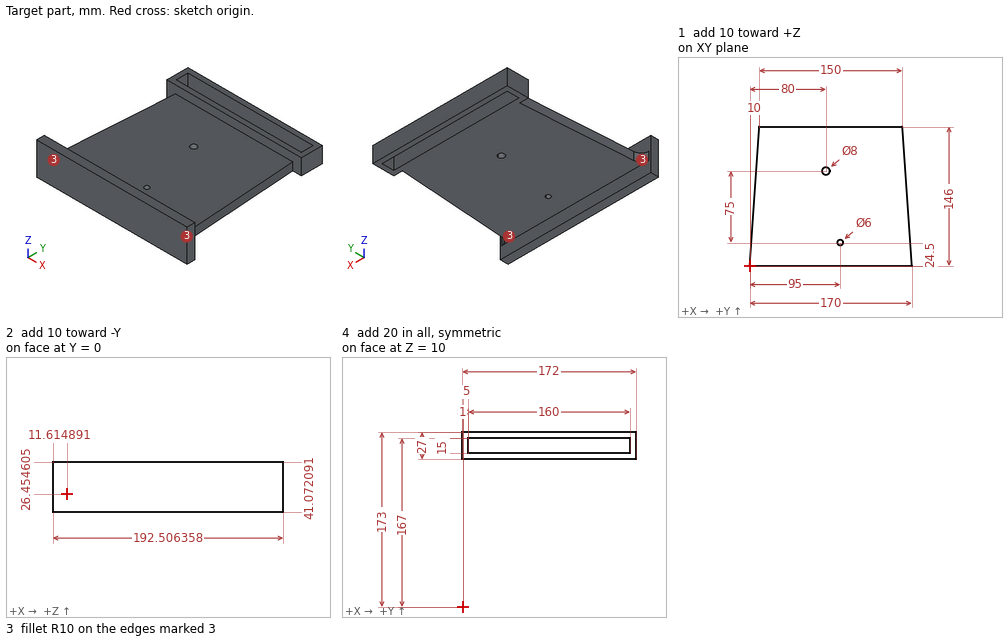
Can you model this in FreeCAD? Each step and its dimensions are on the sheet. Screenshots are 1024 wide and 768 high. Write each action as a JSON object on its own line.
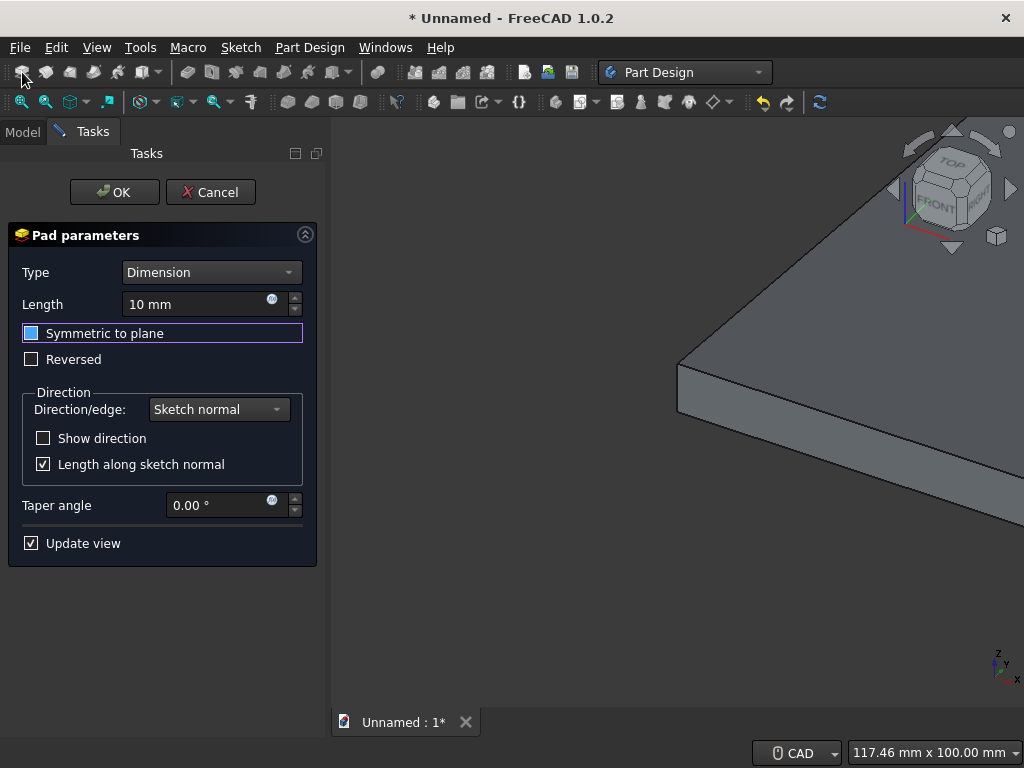
{"action": "left_click", "coordinate": [115, 192]}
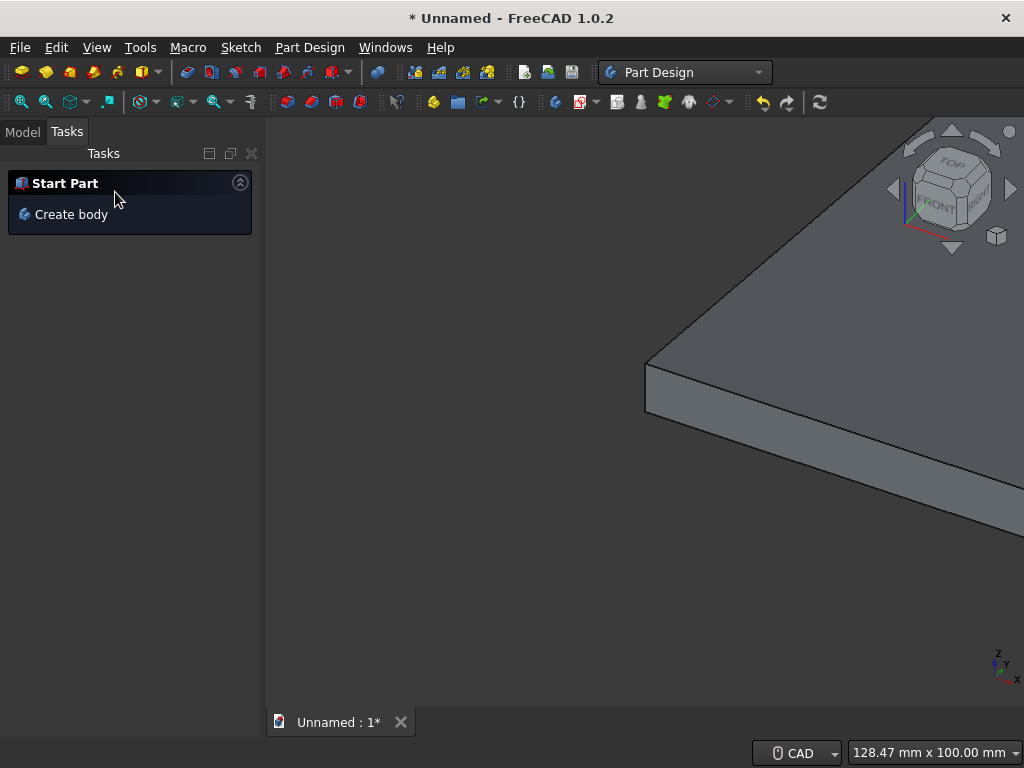
{"action": "key", "text": "v f"}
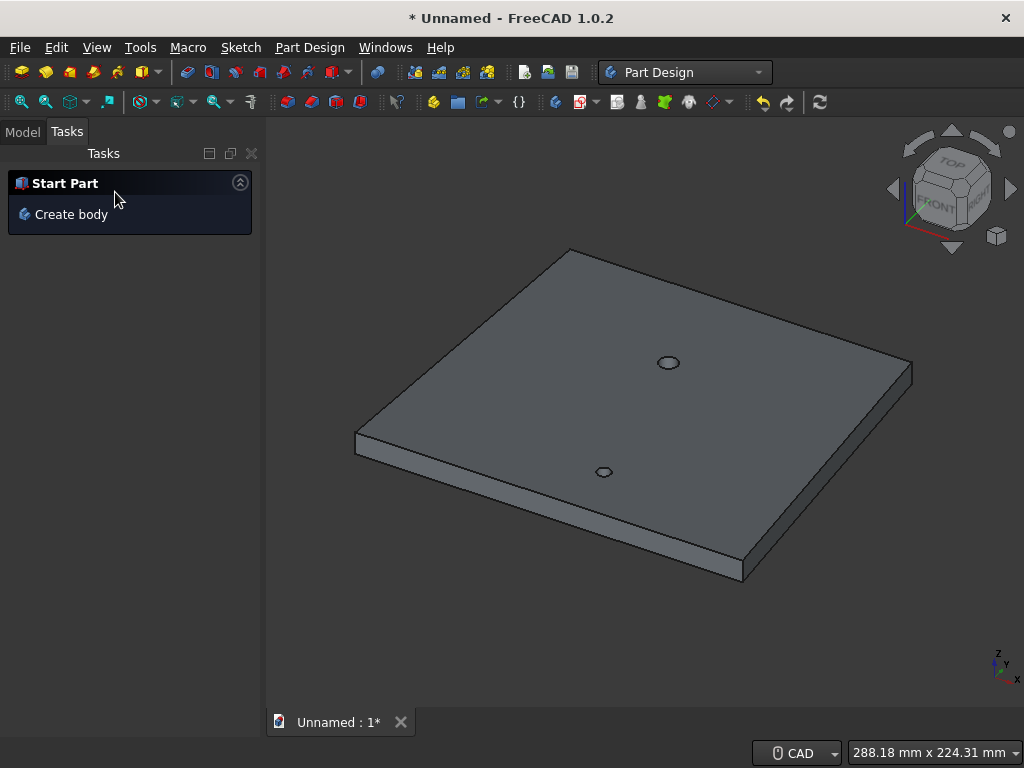
{"action": "left_click", "coordinate": [715, 561]}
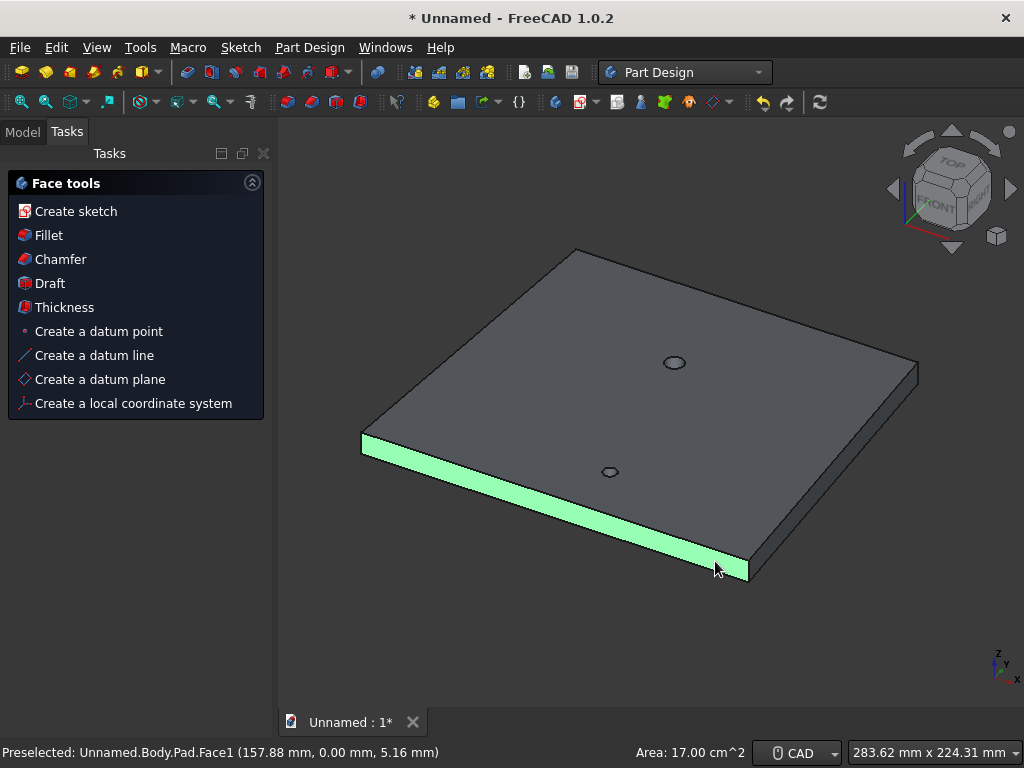
{"action": "left_click", "coordinate": [580, 102]}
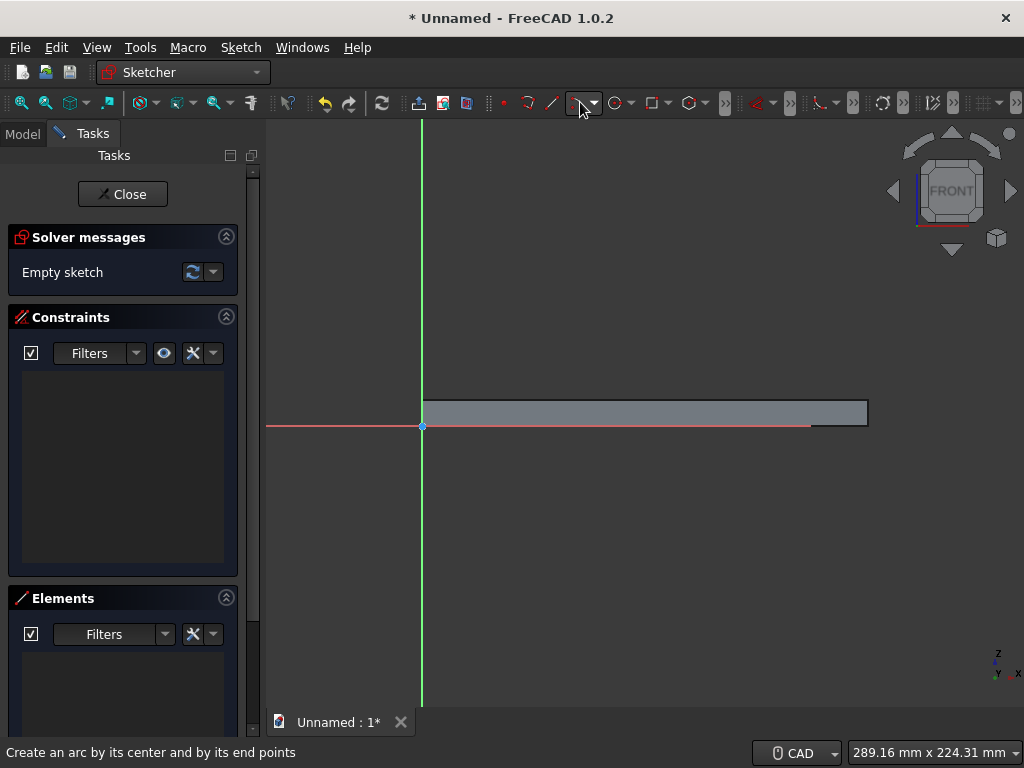
{"action": "scroll", "coordinate": [294, 424], "scroll_direction": "down", "scroll_amount": 1}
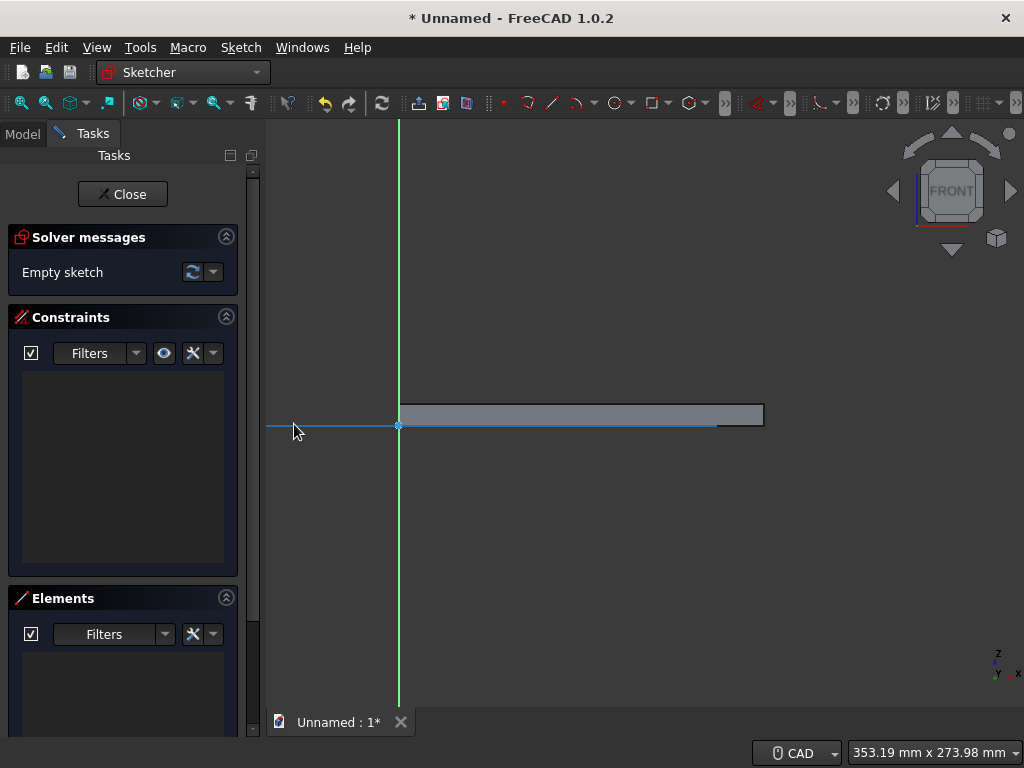
{"action": "key", "text": "g r"}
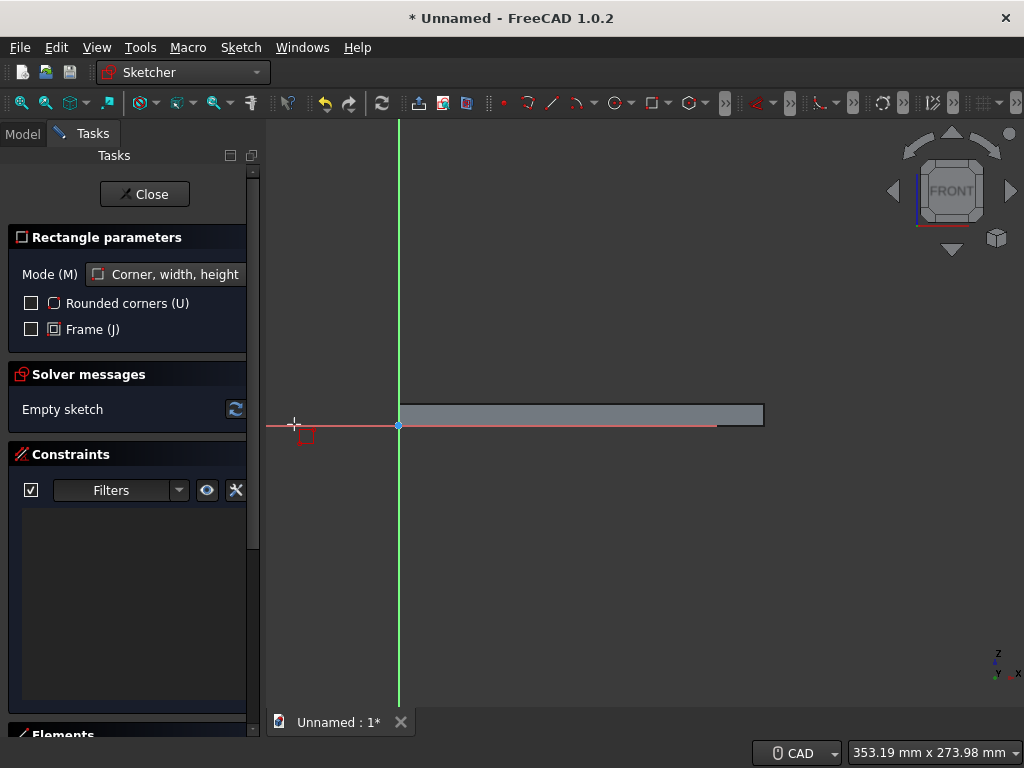
{"action": "left_click", "coordinate": [374, 369]}
{"action": "mouse_move", "coordinate": [787, 457]}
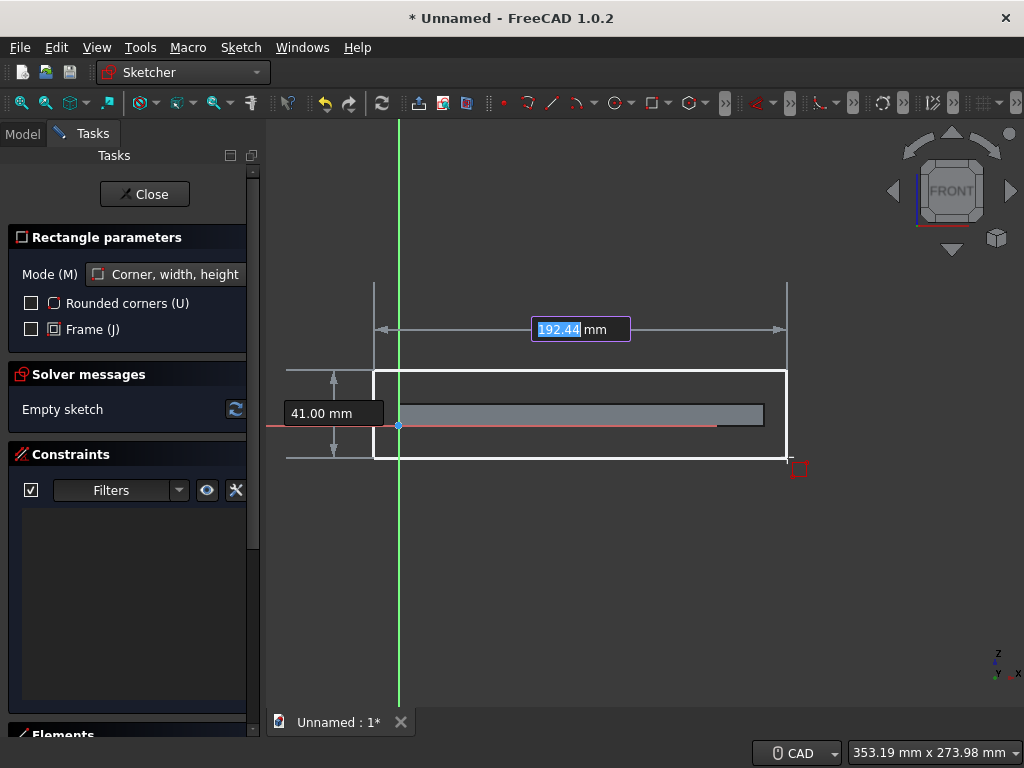
{"action": "type", "text": "192.506358"}
{"action": "key", "text": "Tab"}
{"action": "type", "text": "41.072091"}
{"action": "key", "text": "Return"}
{"action": "key", "text": "Escape"}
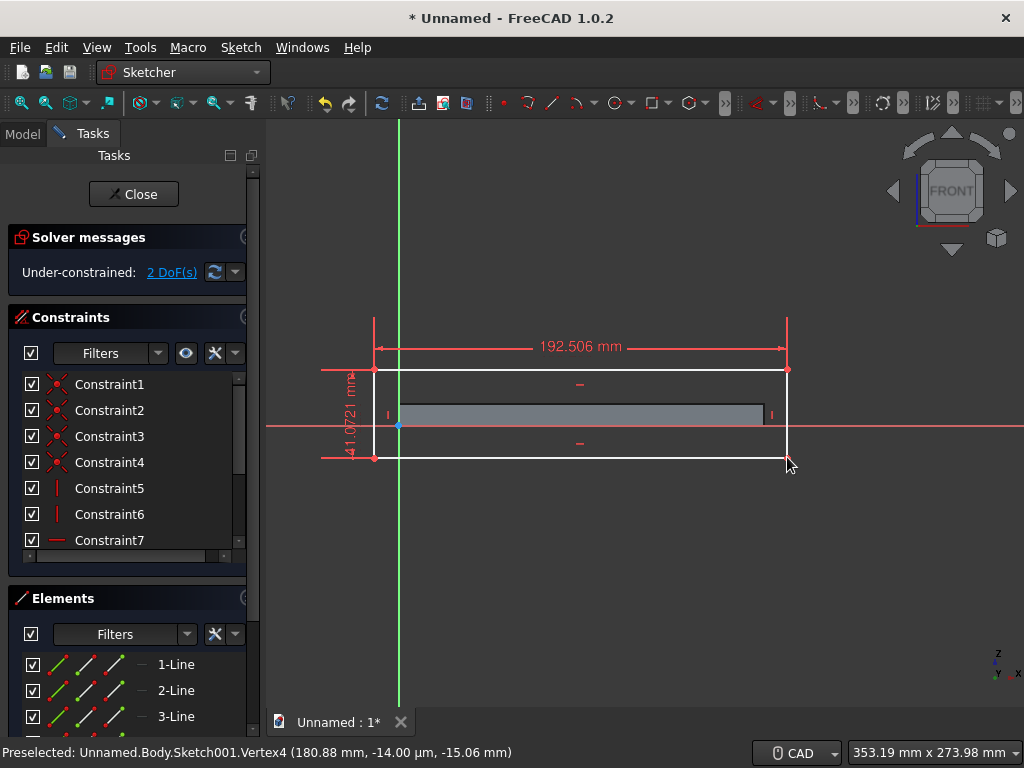
{"action": "key", "text": "d"}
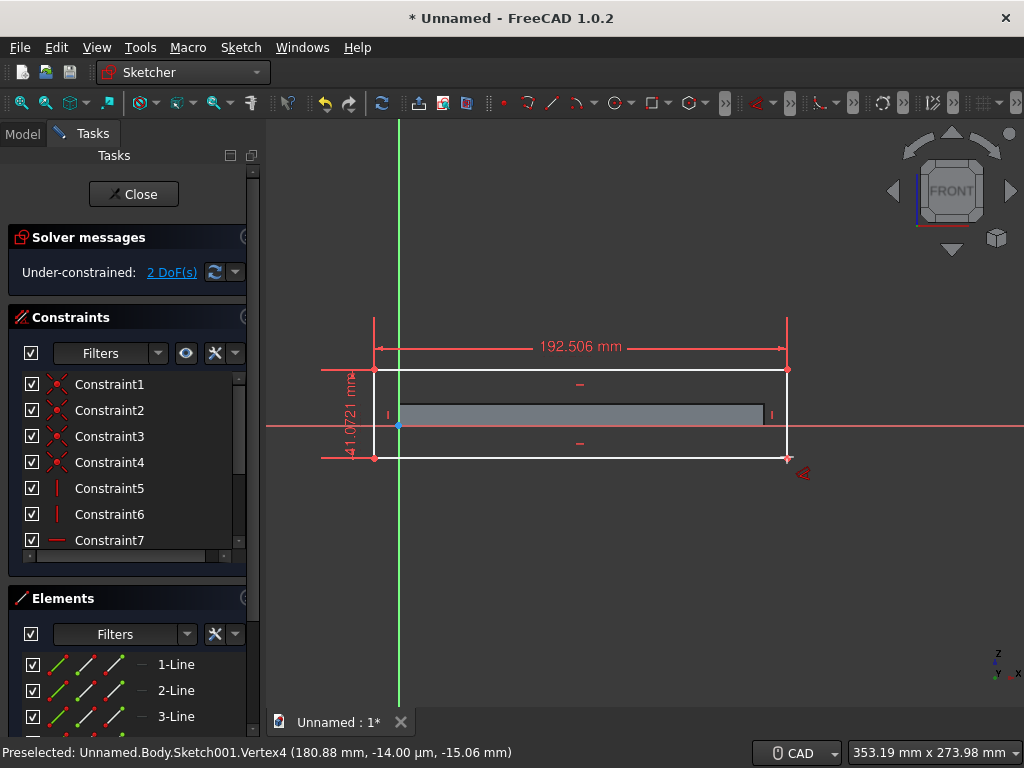
{"action": "scroll", "coordinate": [374, 370], "scroll_direction": "up", "scroll_amount": 3}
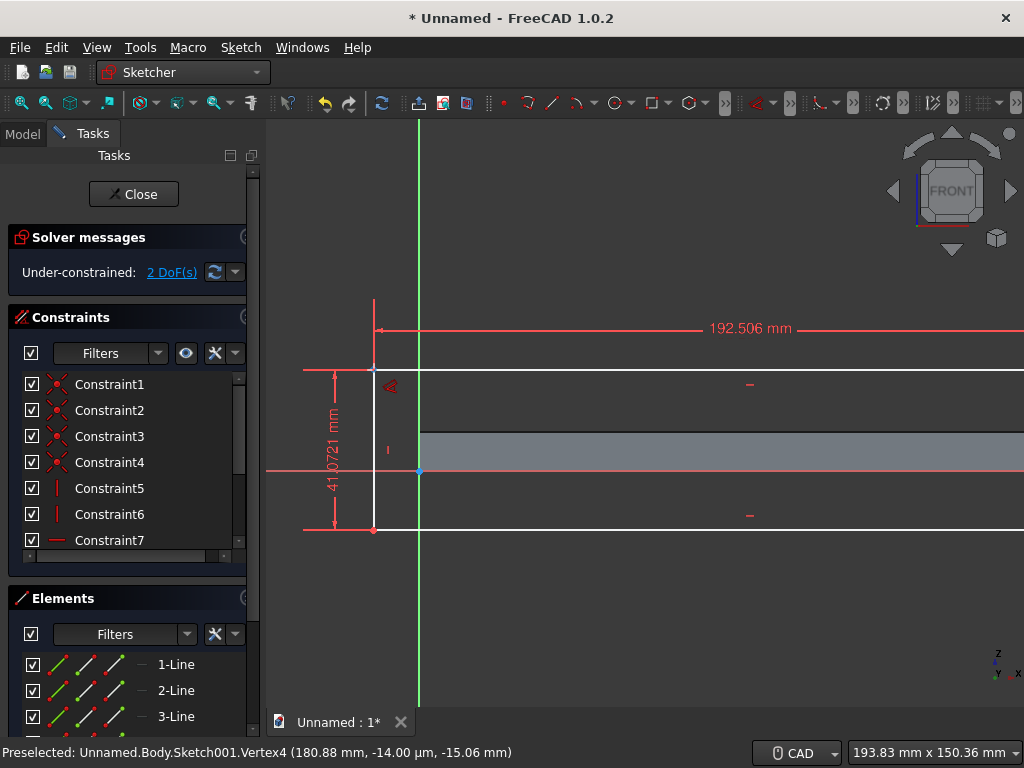
{"action": "left_click", "coordinate": [374, 370]}
{"action": "left_click", "coordinate": [397, 336]}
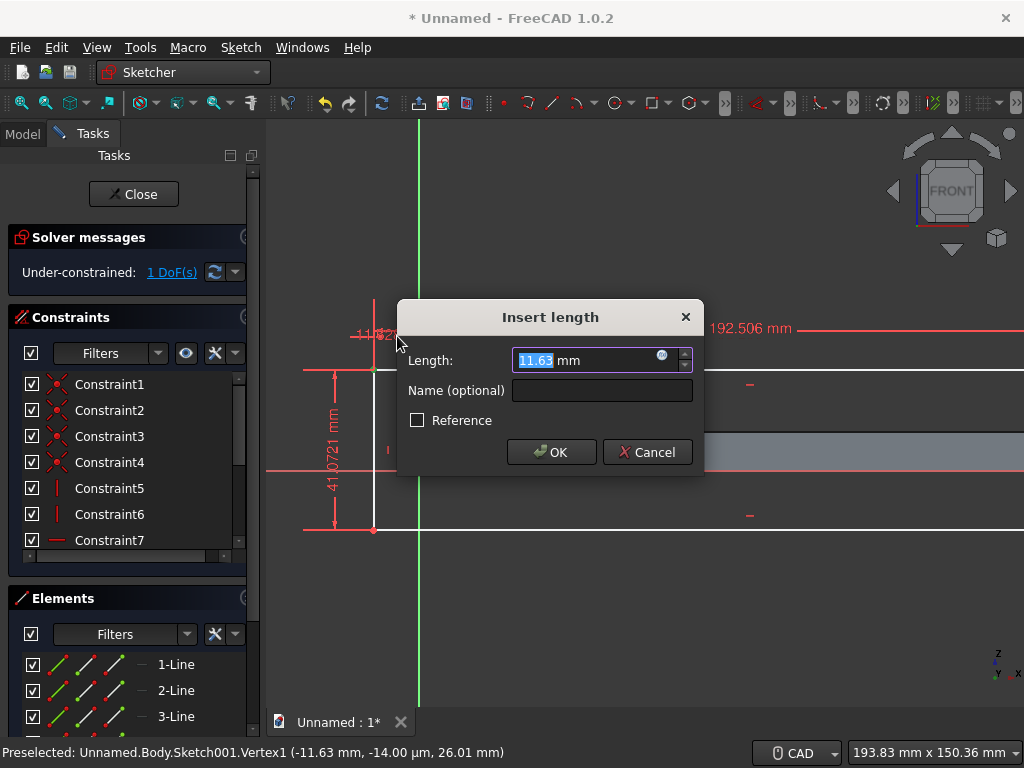
{"action": "type", "text": "11.614891"}
{"action": "key", "text": "Return"}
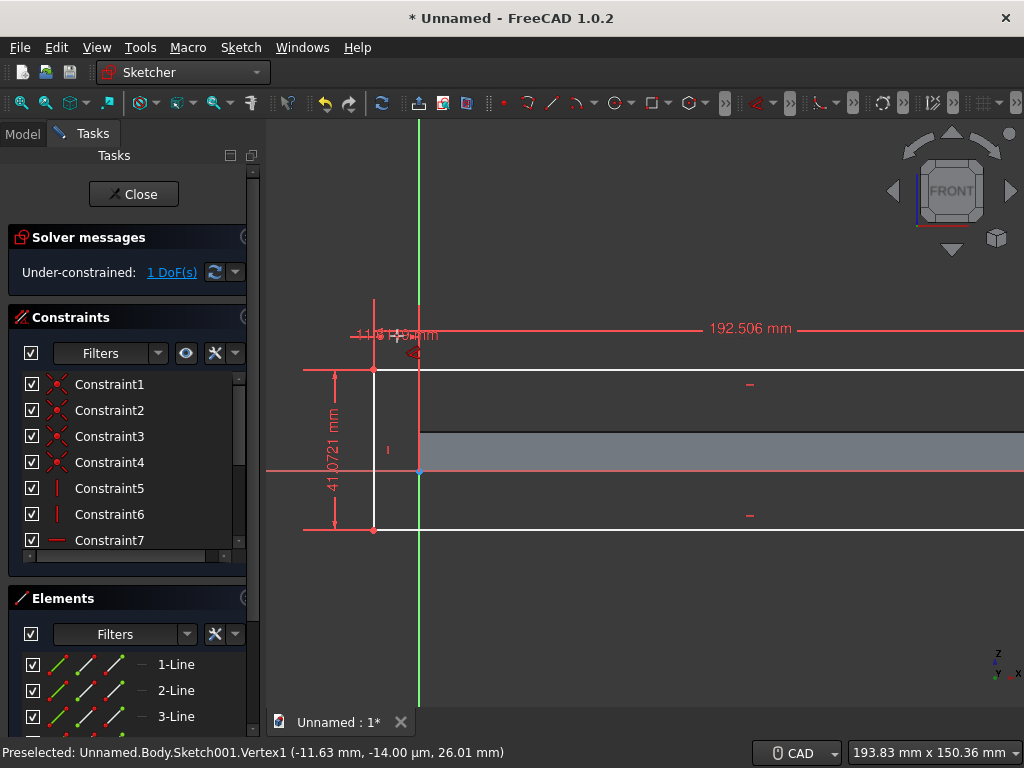
{"action": "left_click", "coordinate": [374, 370]}
{"action": "left_click", "coordinate": [340, 421]}